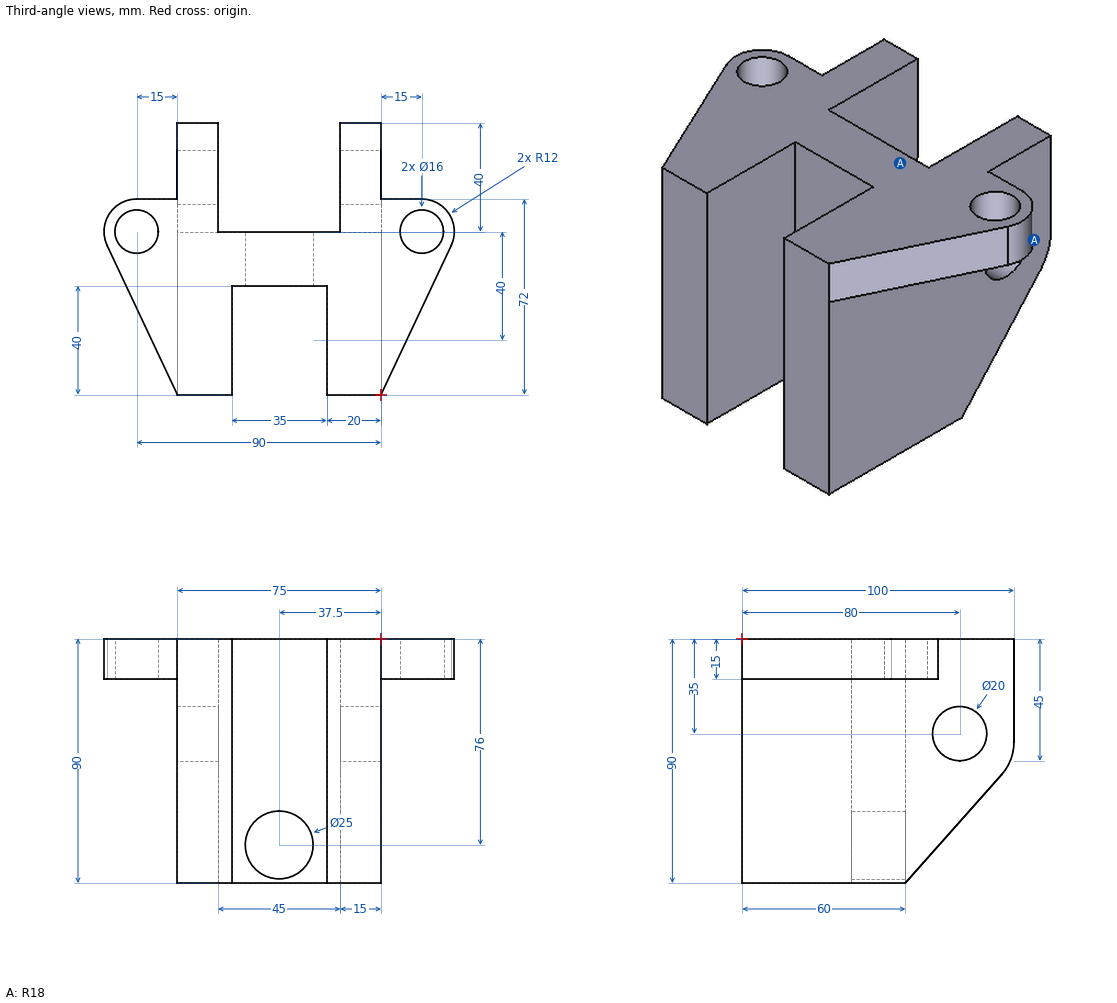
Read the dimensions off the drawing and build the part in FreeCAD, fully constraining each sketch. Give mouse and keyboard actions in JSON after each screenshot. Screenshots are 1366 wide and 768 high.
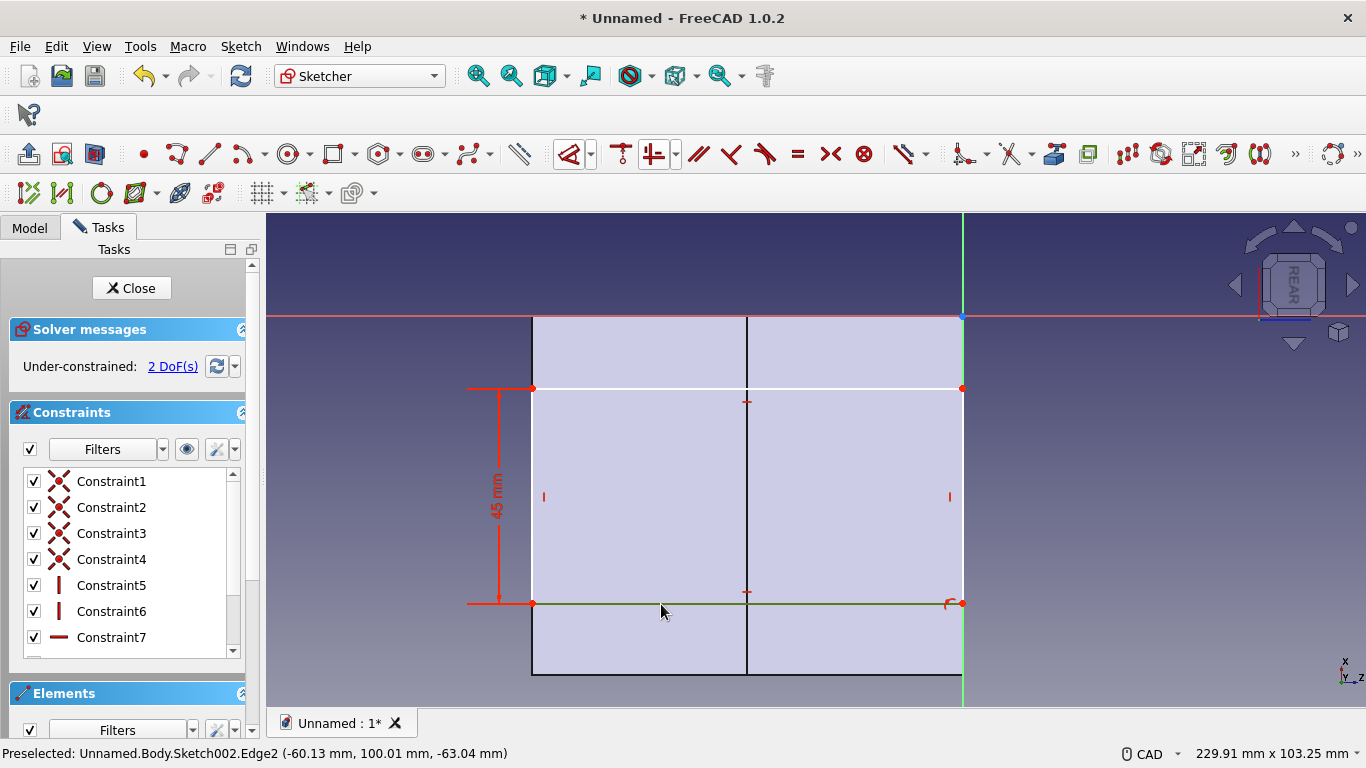
{"action": "key", "text": "l"}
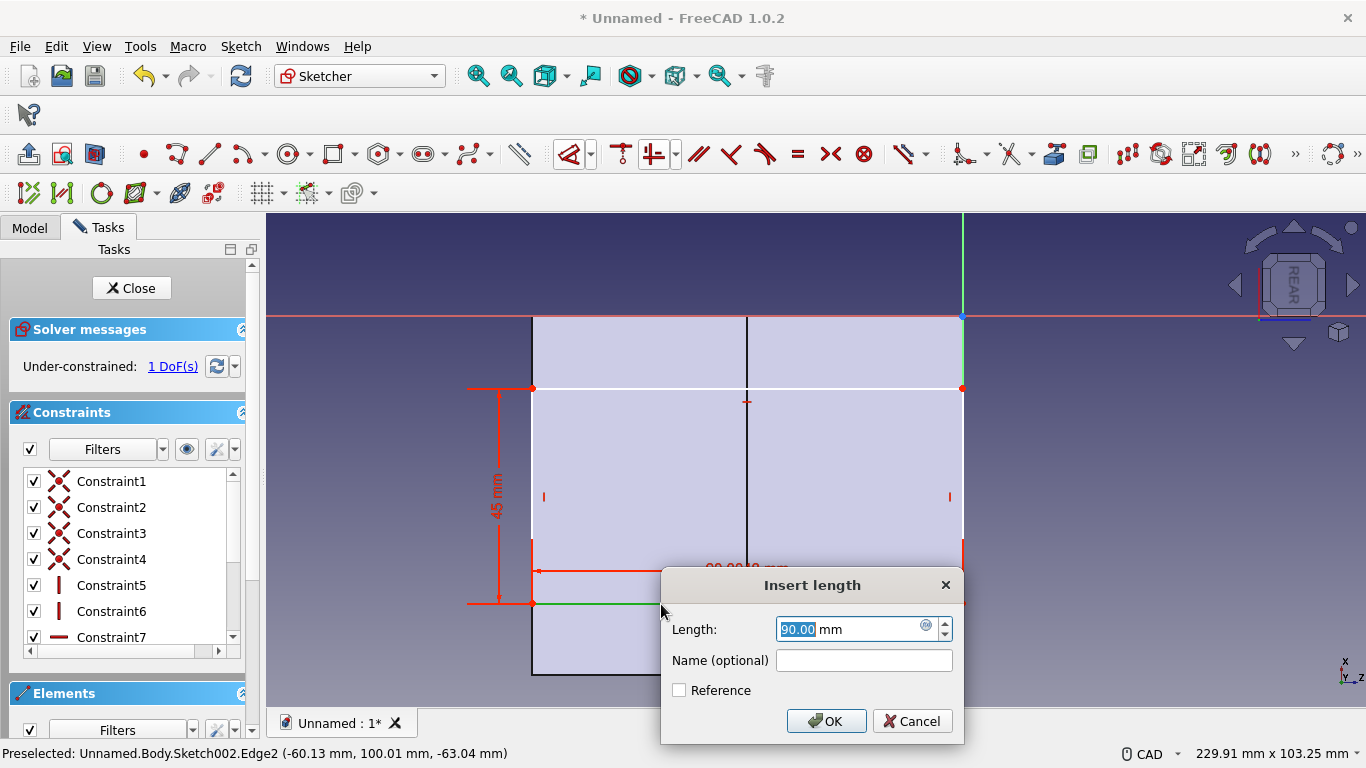
{"action": "type", "text": "90"}
{"action": "key", "text": "Return"}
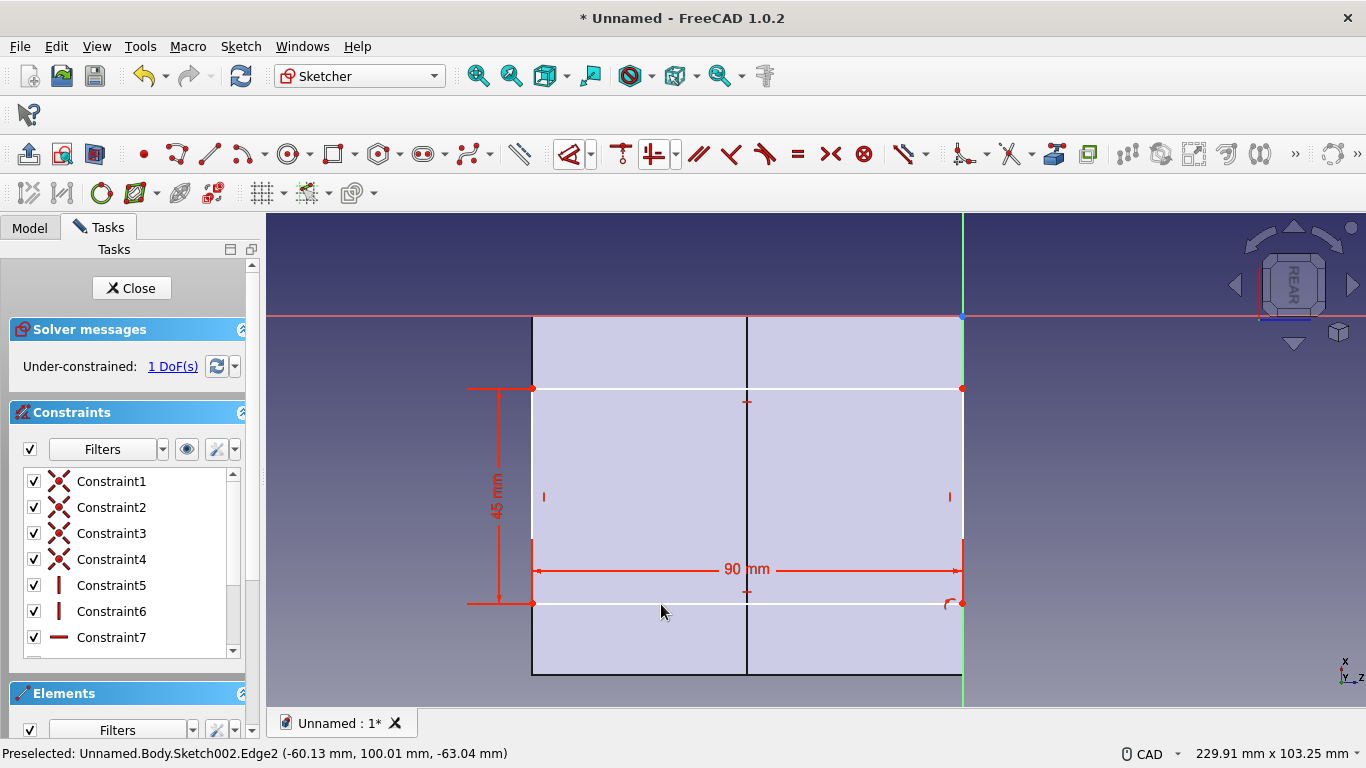
{"action": "left_click", "coordinate": [532, 389]}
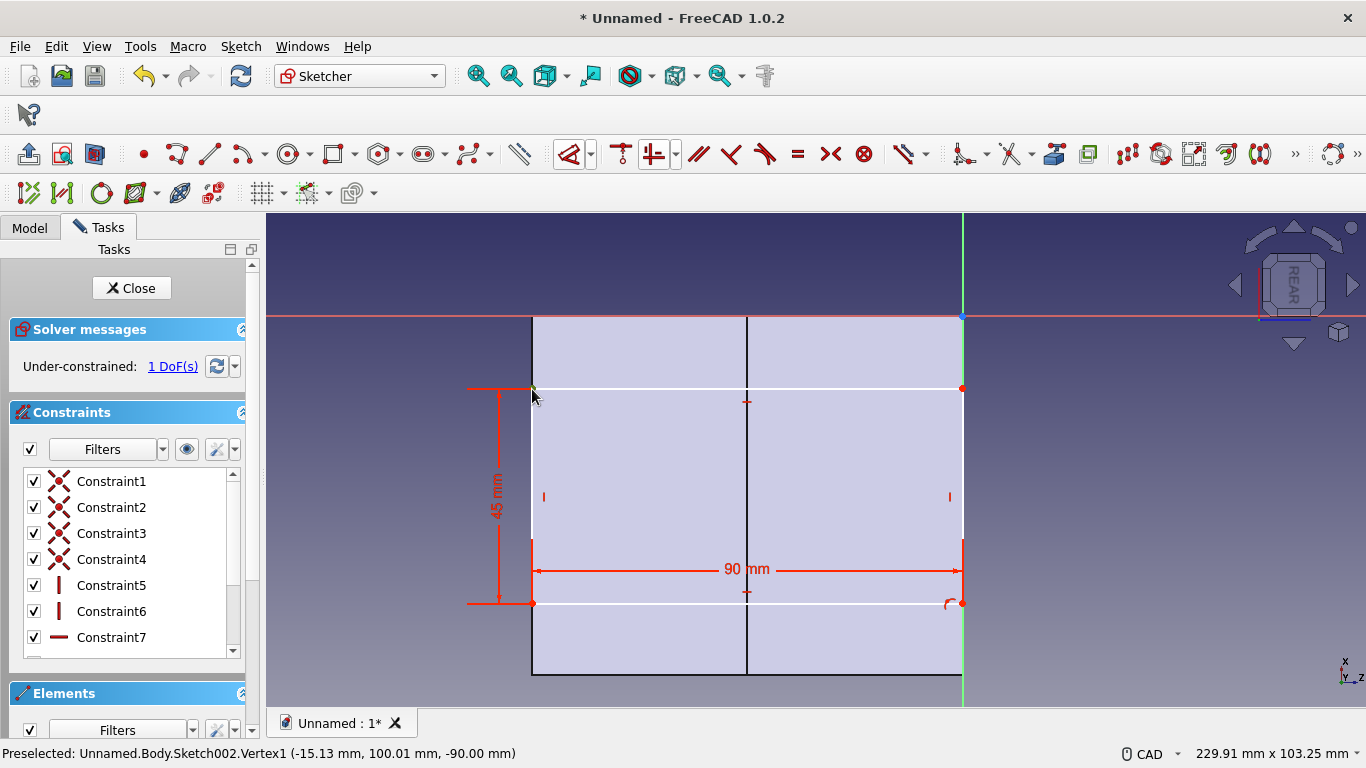
{"action": "key", "text": "i"}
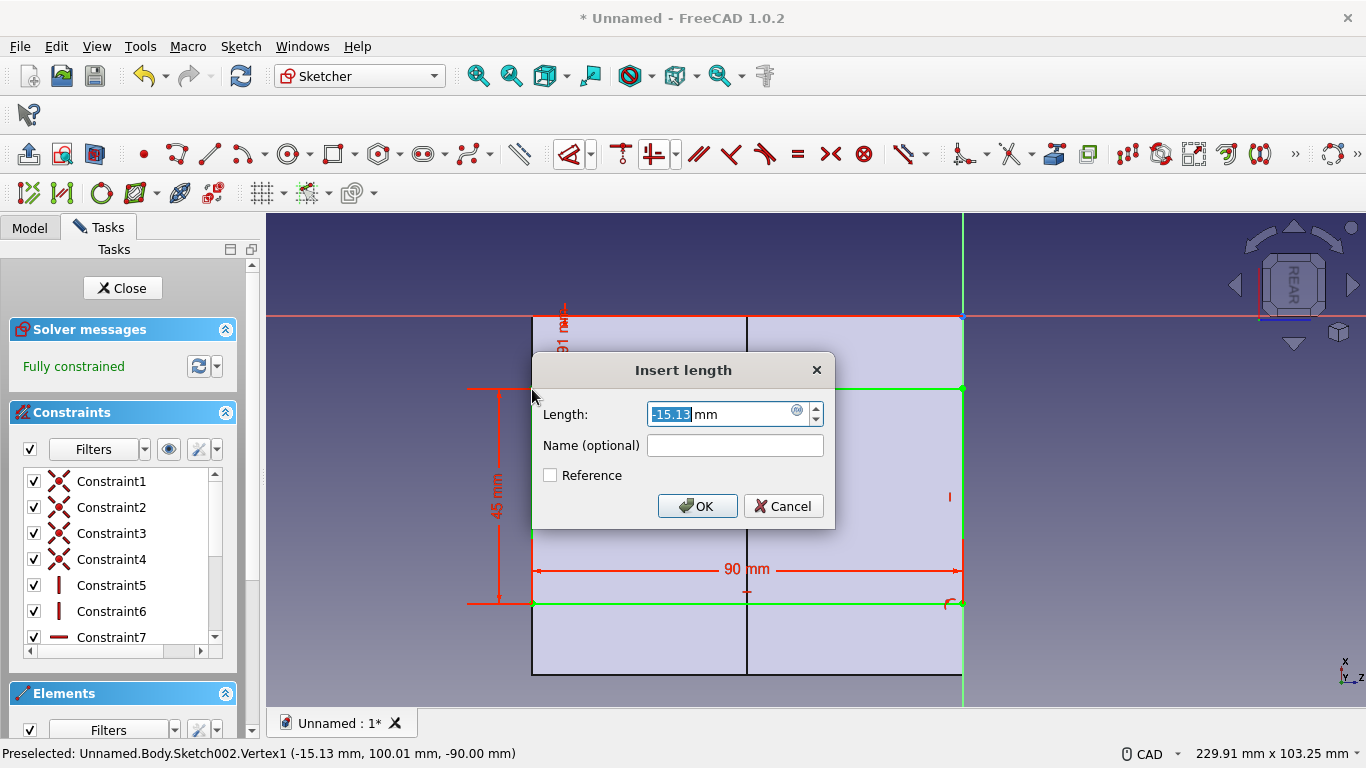
{"action": "type", "text": "-15"}
{"action": "key", "text": "Return"}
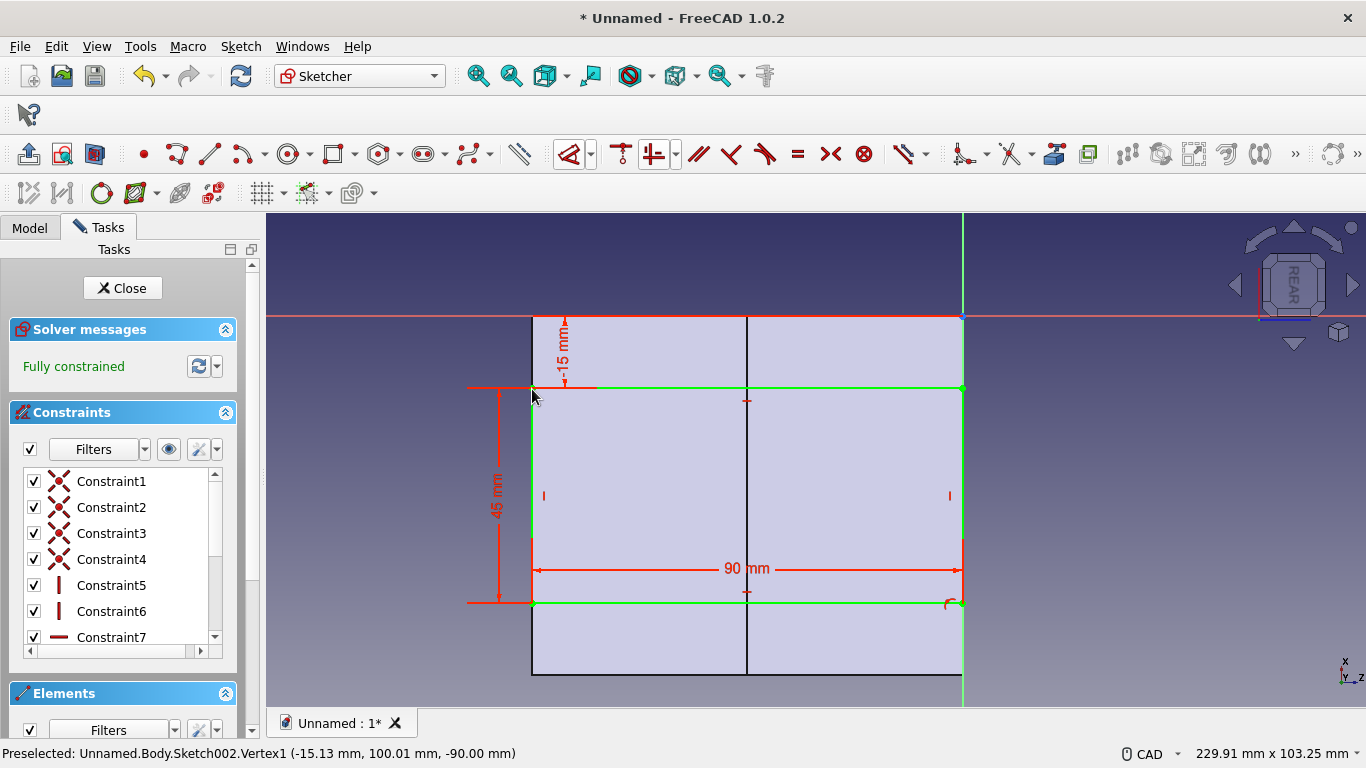
{"action": "left_click", "coordinate": [123, 288]}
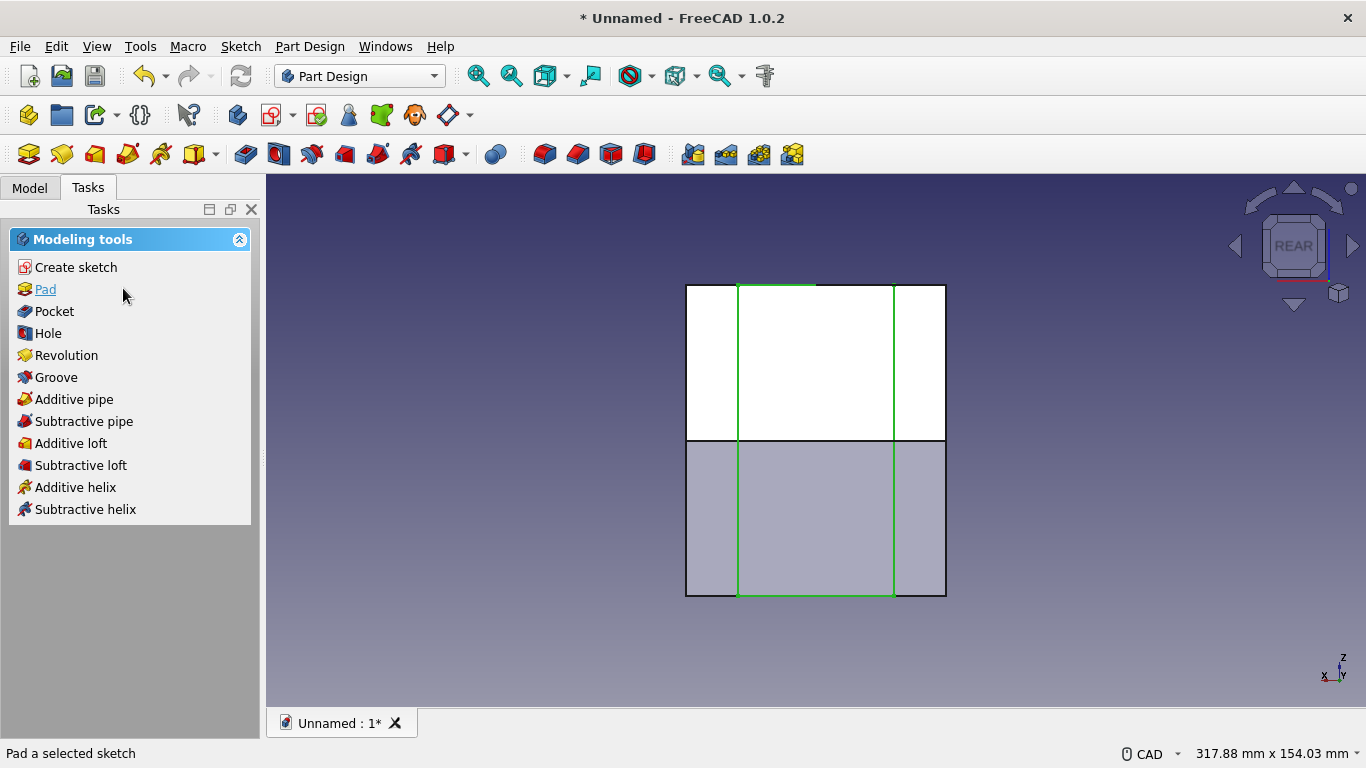
{"action": "left_click", "coordinate": [246, 154]}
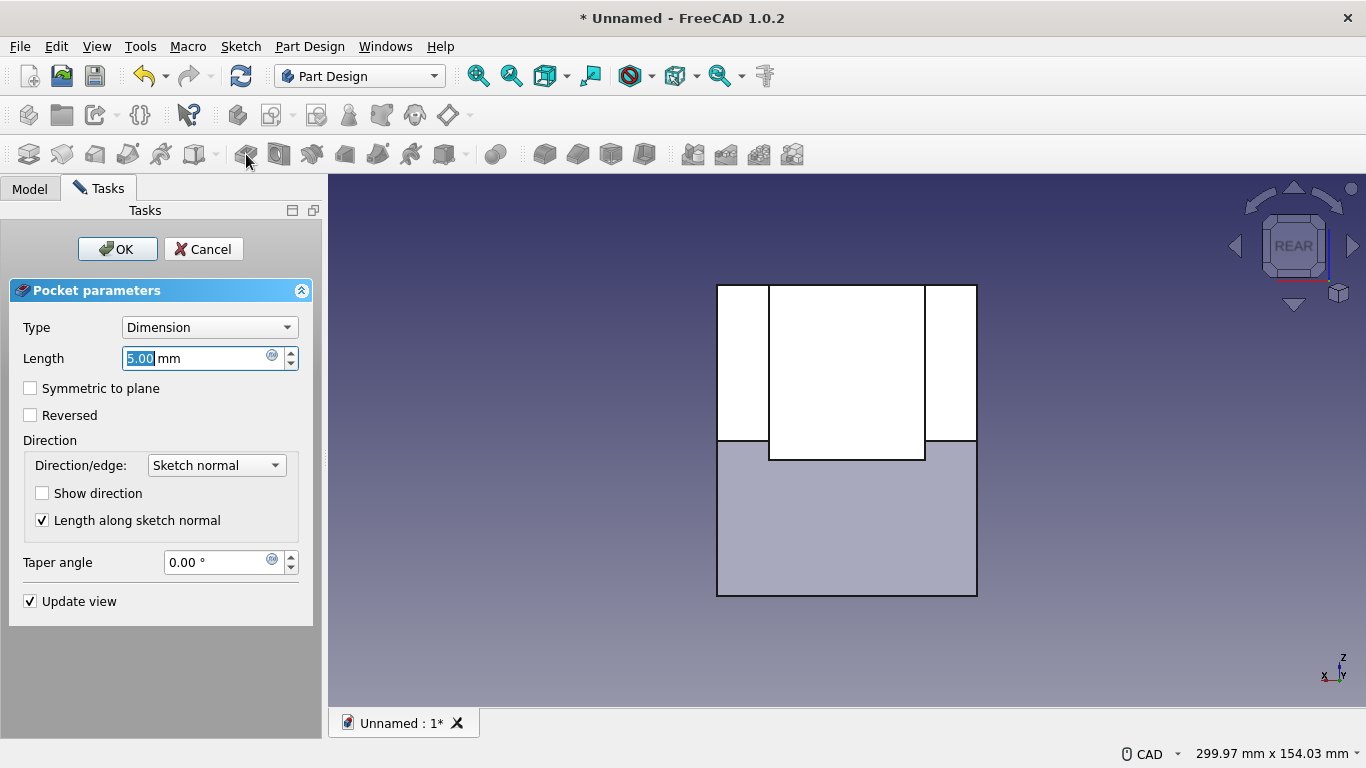
{"action": "type", "text": "40"}
{"action": "key", "text": "Tab"}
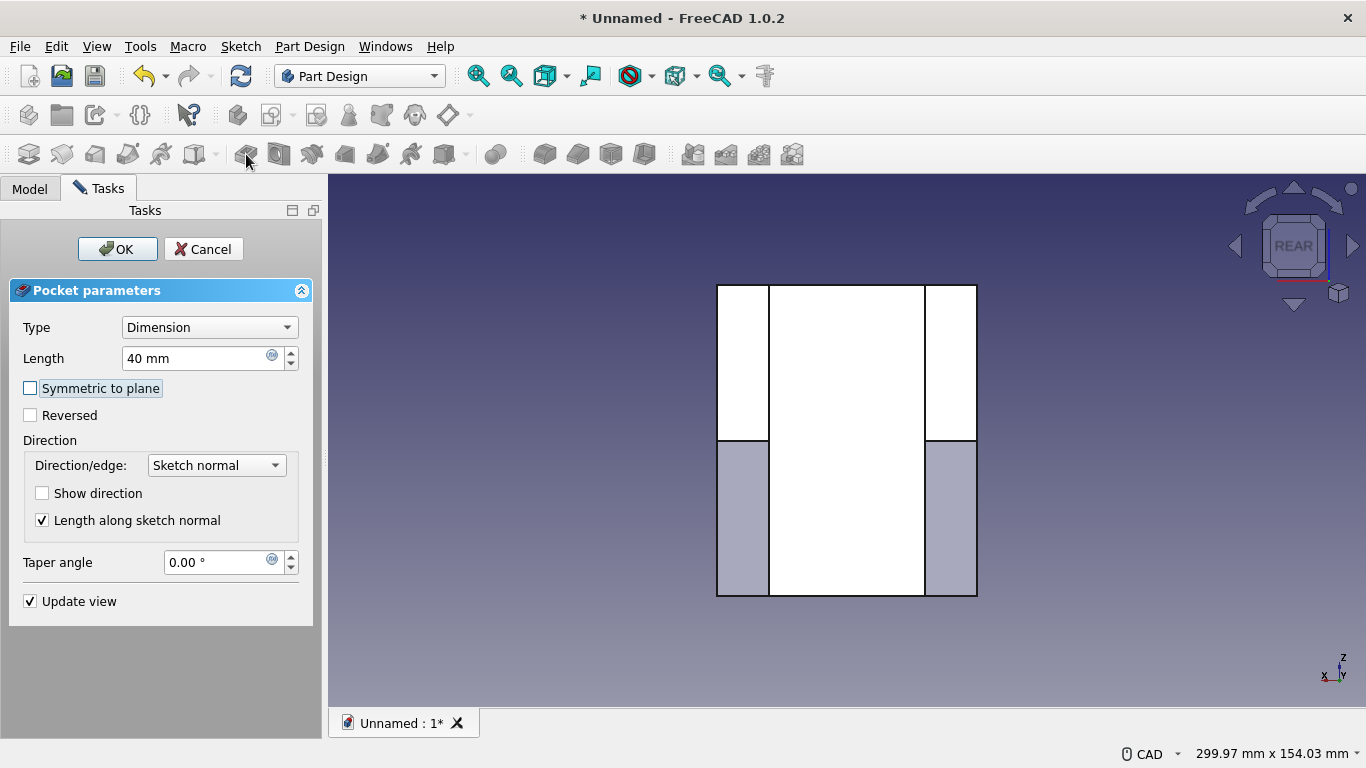
{"action": "left_click", "coordinate": [118, 249]}